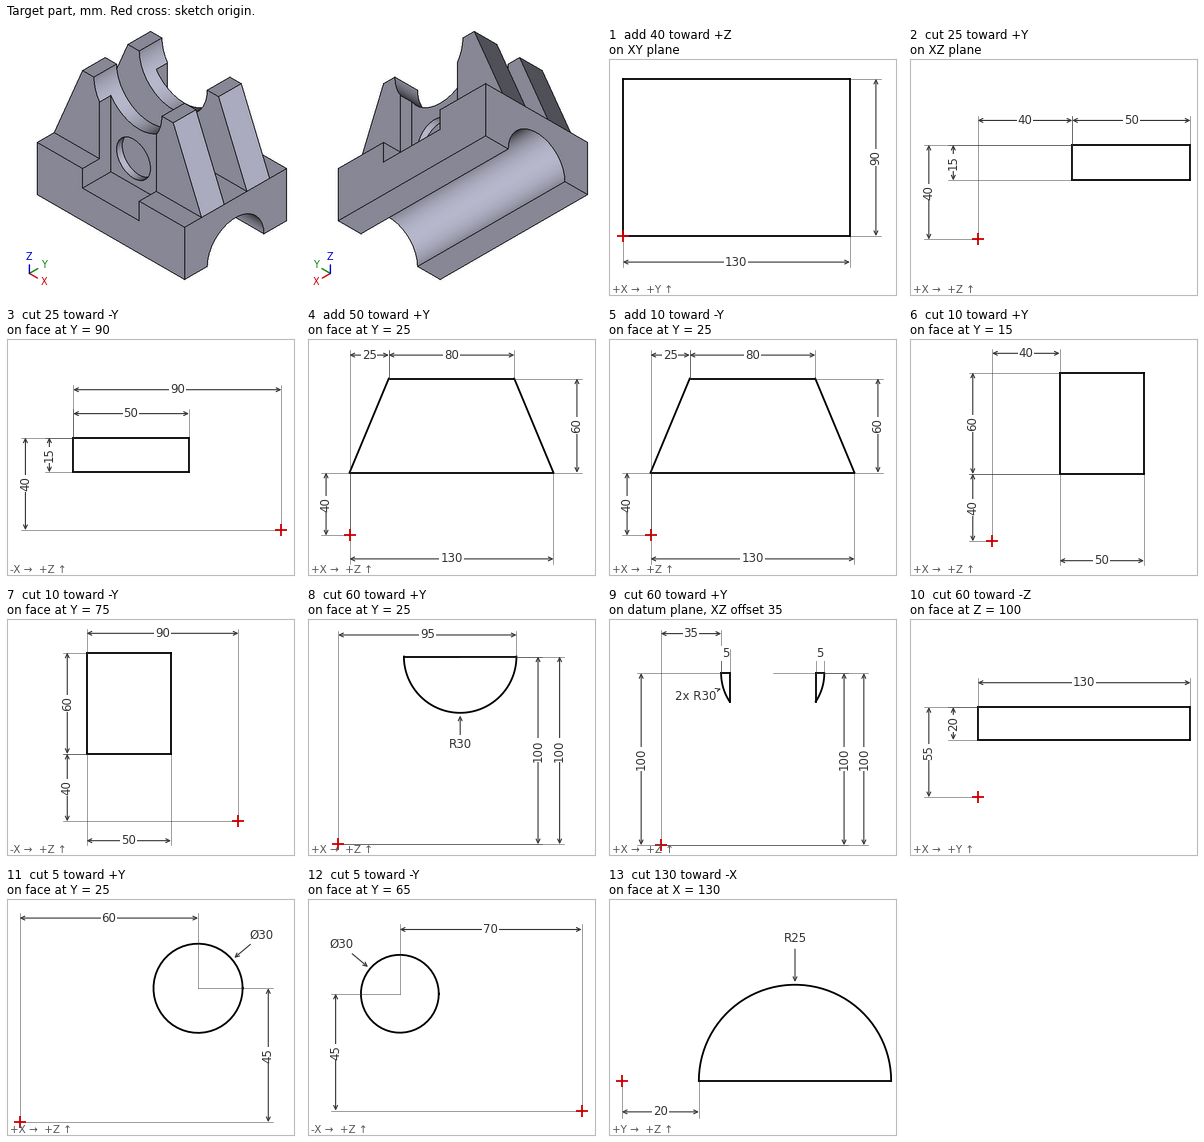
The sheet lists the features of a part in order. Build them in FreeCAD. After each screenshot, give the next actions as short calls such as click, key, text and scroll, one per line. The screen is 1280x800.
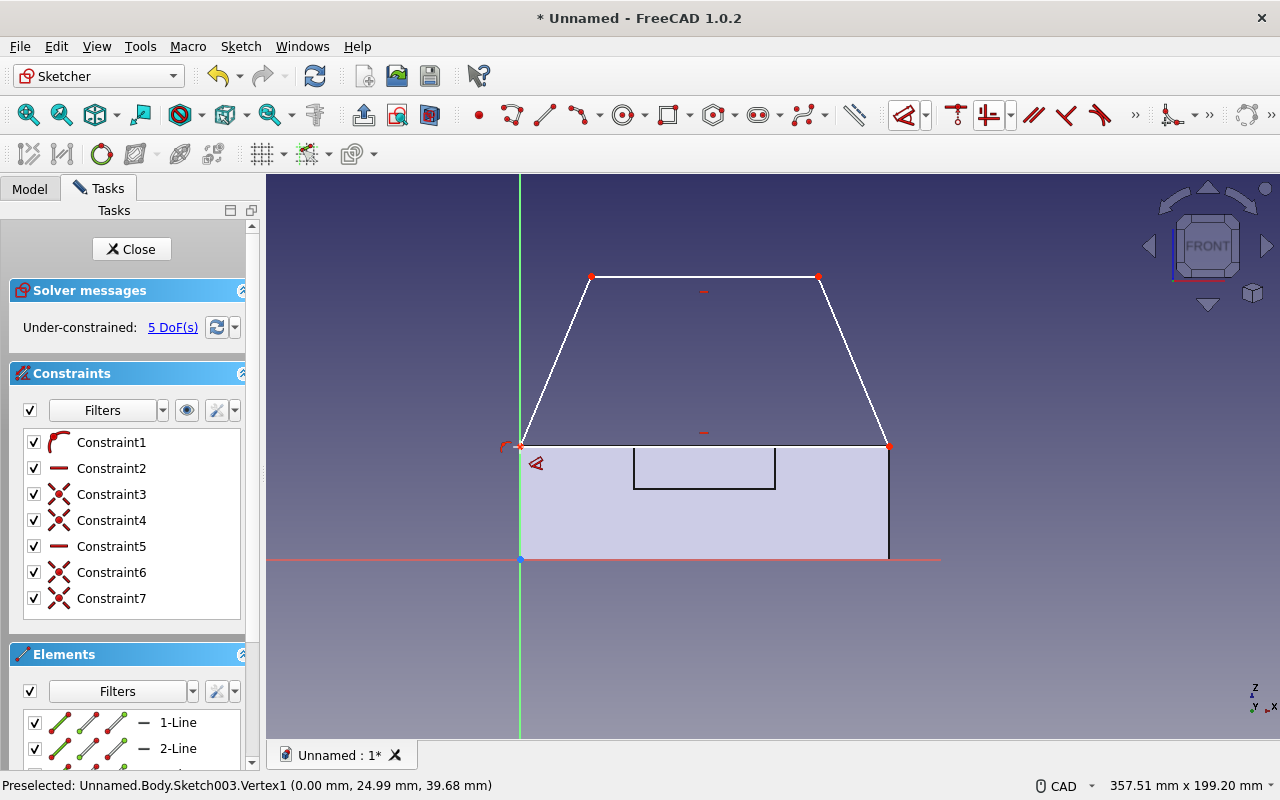
click(750, 277)
click(704, 243)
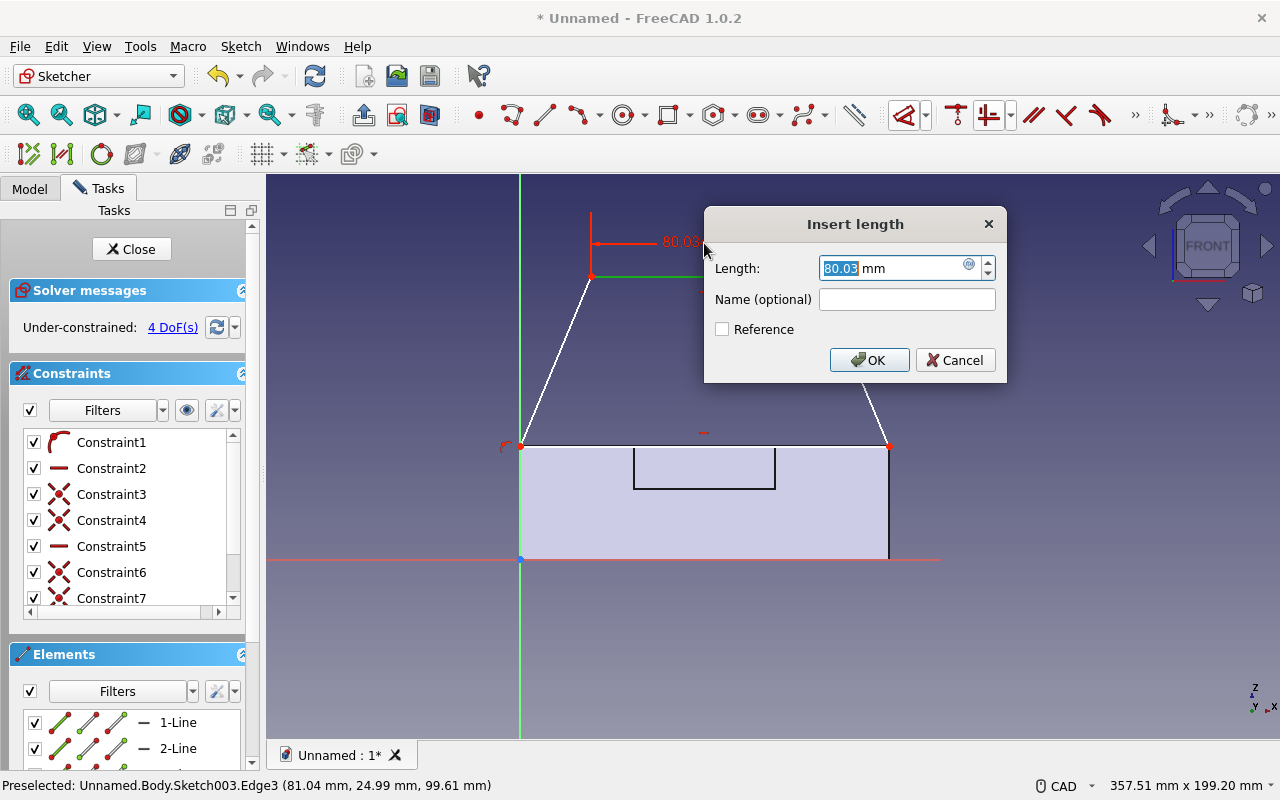
text(80)
key(Return)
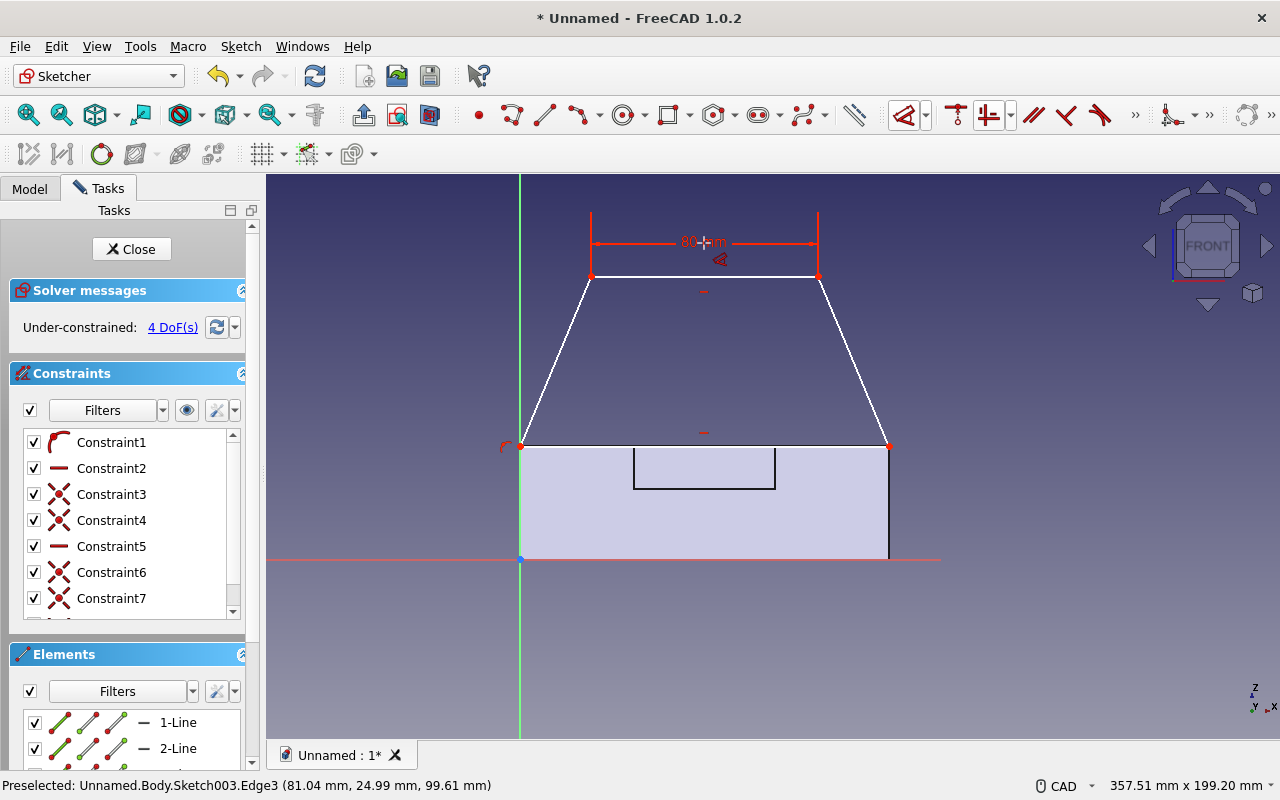
click(631, 447)
click(705, 481)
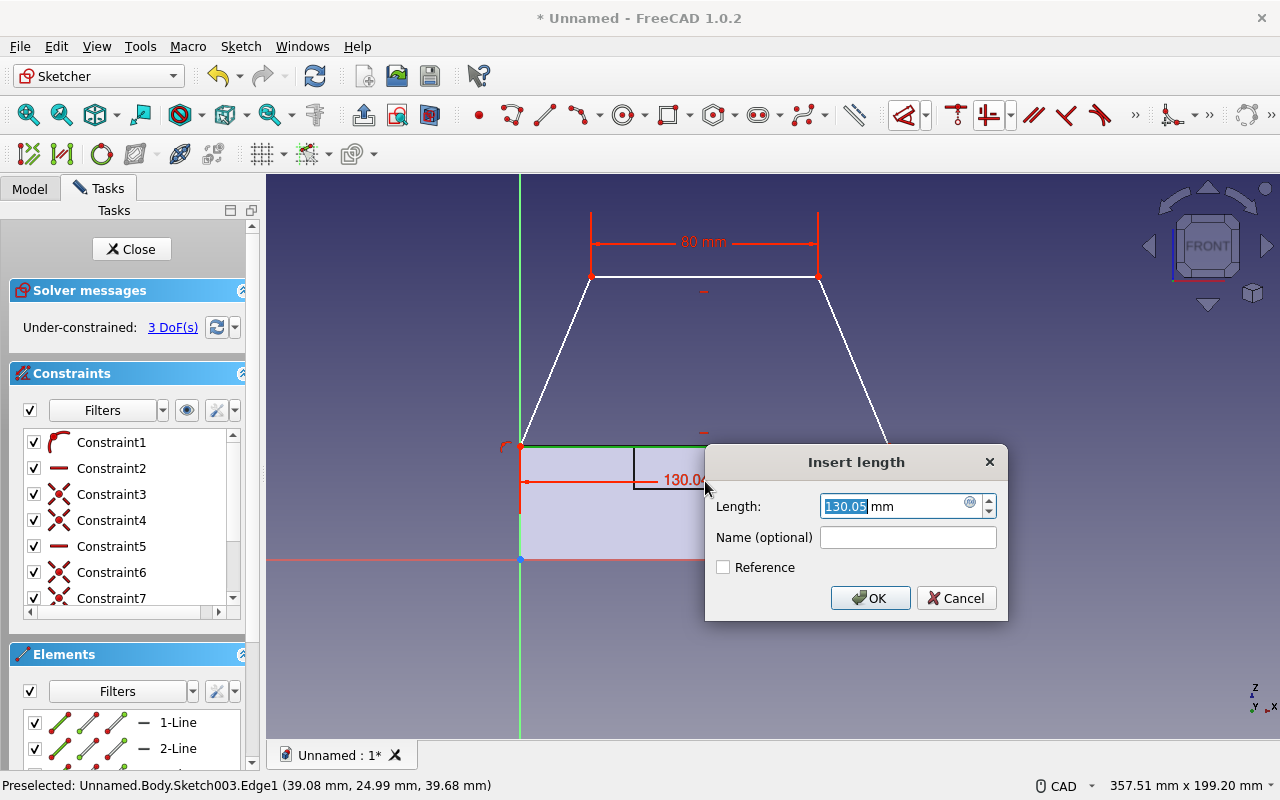
text(130)
key(Return)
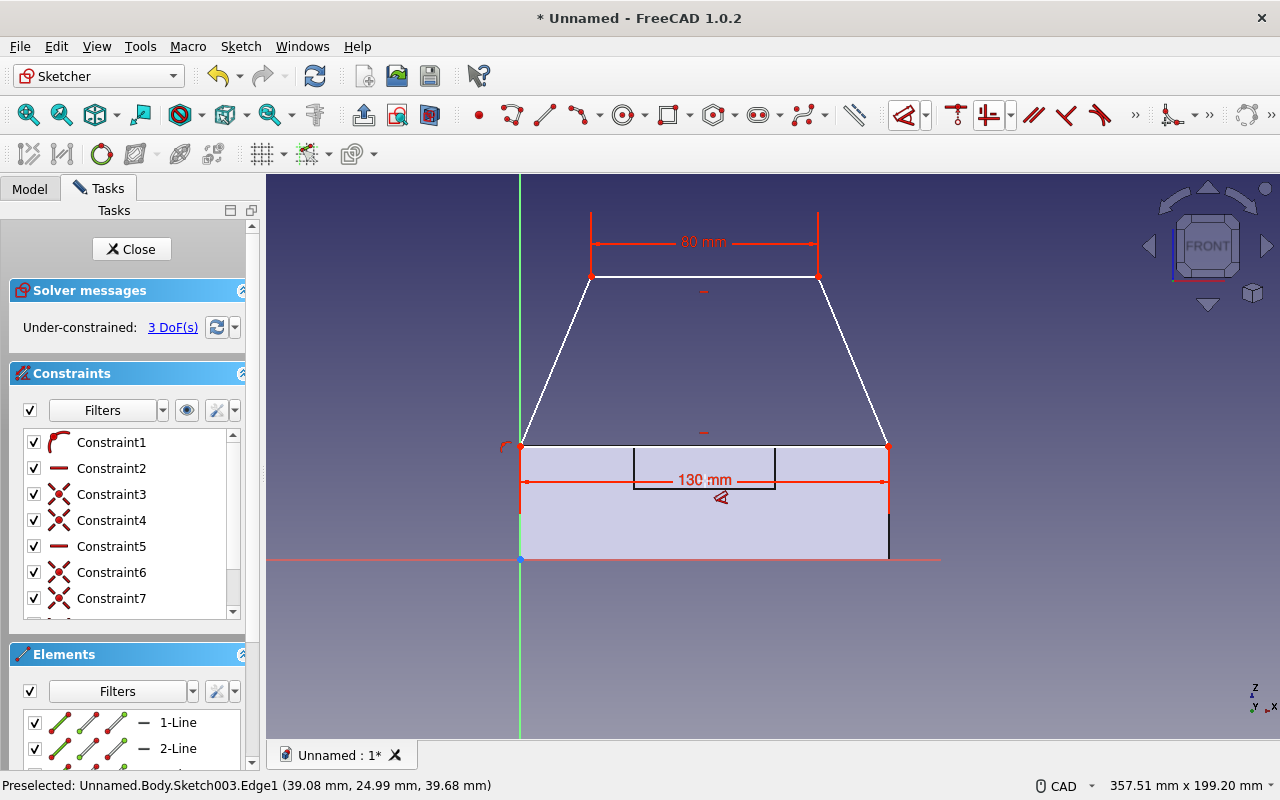
click(520, 447)
click(486, 503)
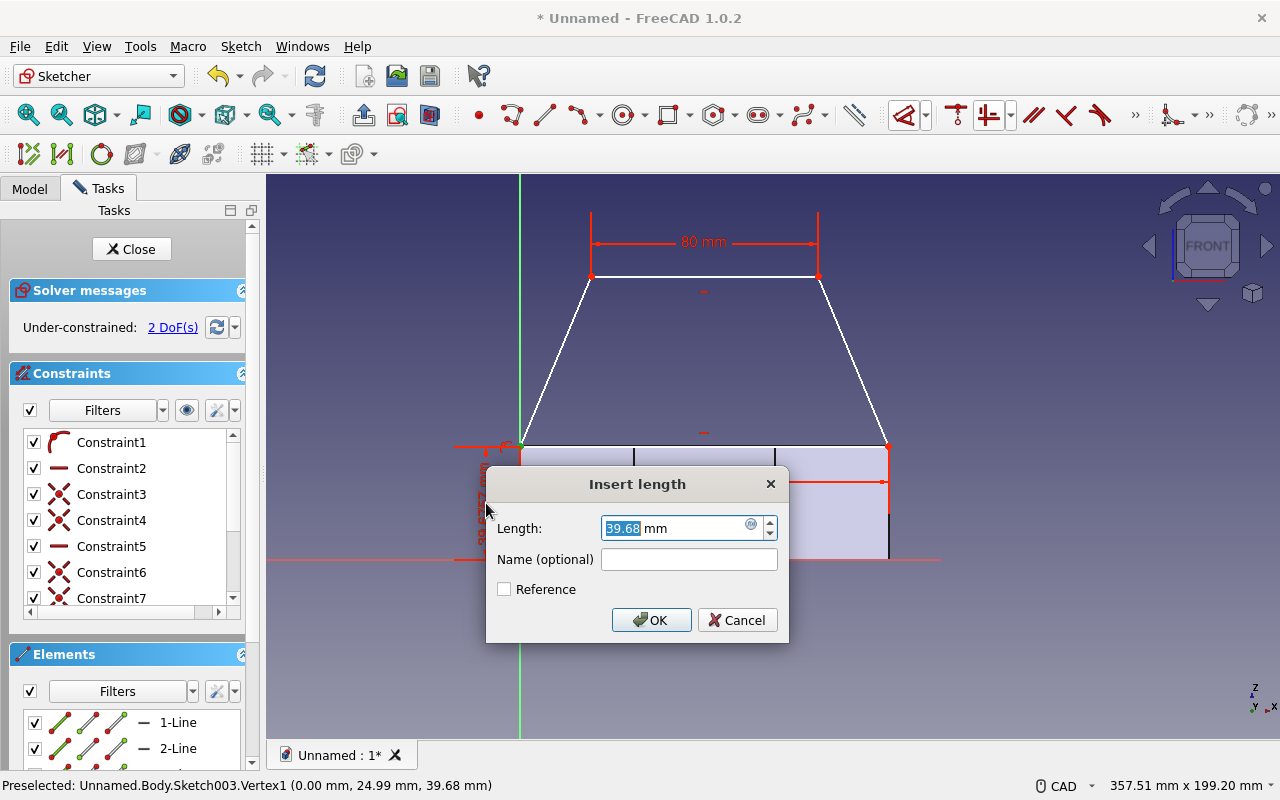
text(40)
key(Return)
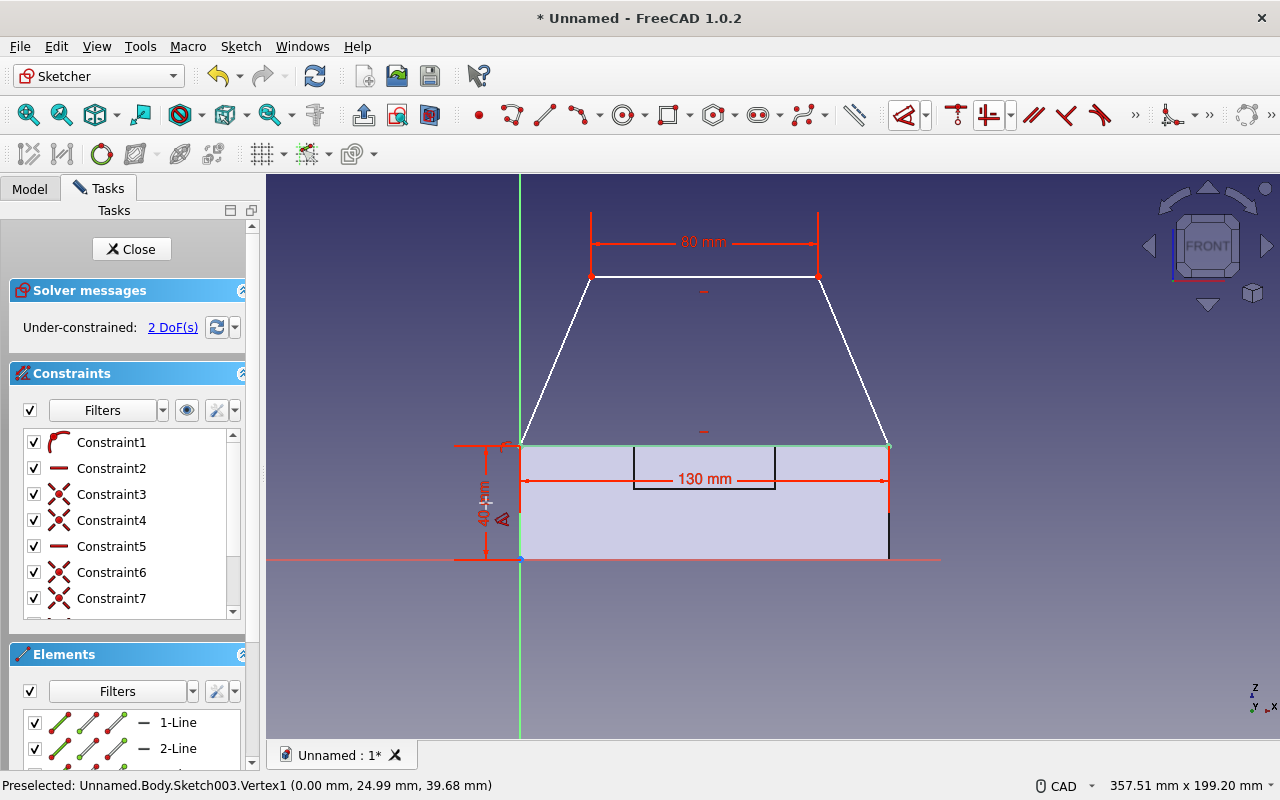
click(591, 277)
click(556, 594)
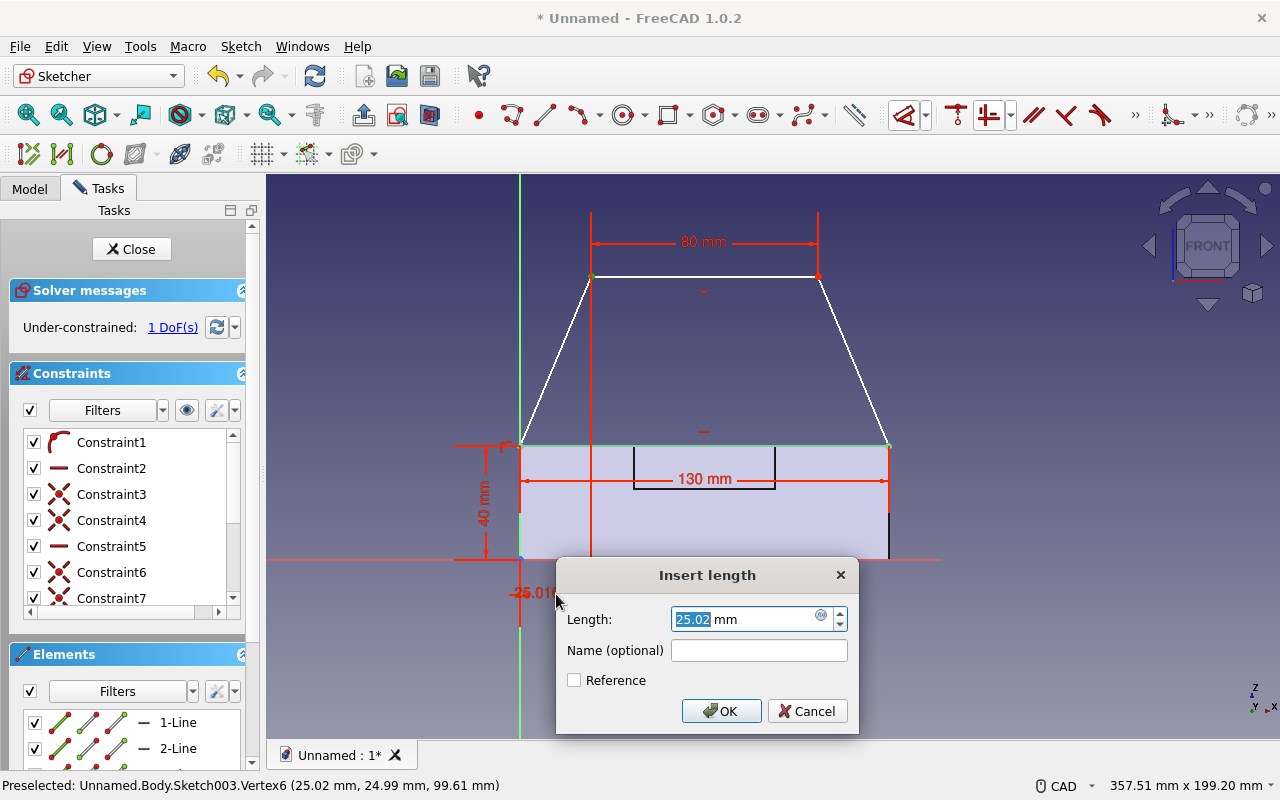
text(25)
key(Return)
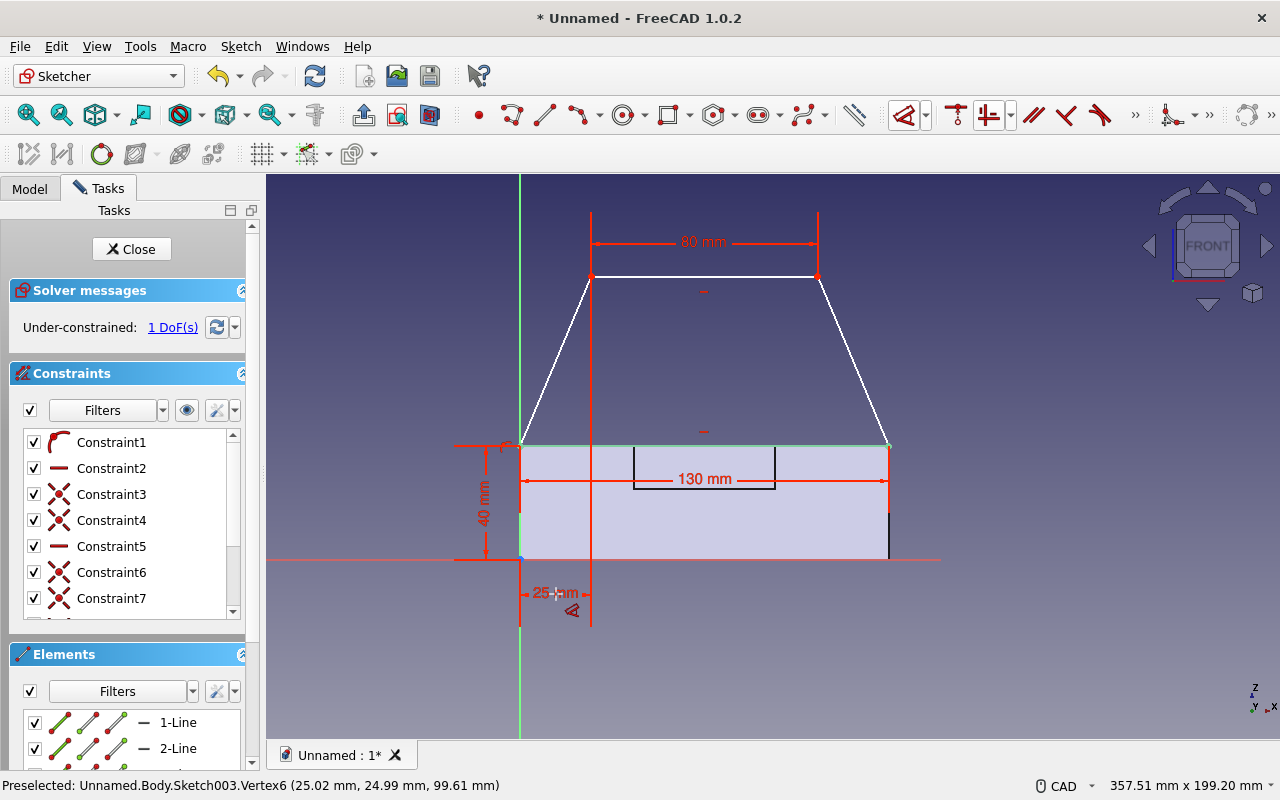
click(868, 395)
click(923, 362)